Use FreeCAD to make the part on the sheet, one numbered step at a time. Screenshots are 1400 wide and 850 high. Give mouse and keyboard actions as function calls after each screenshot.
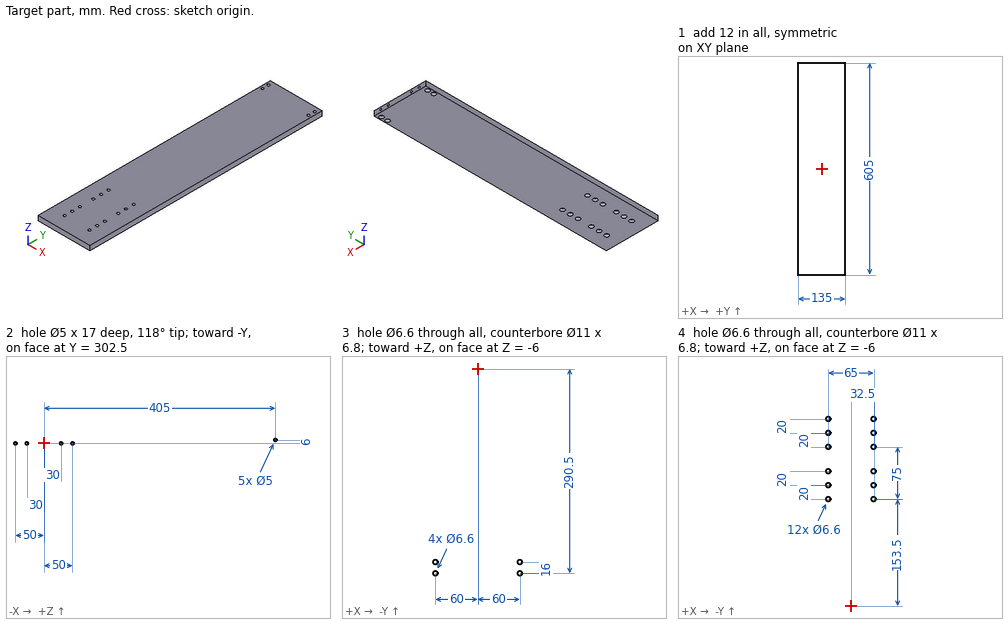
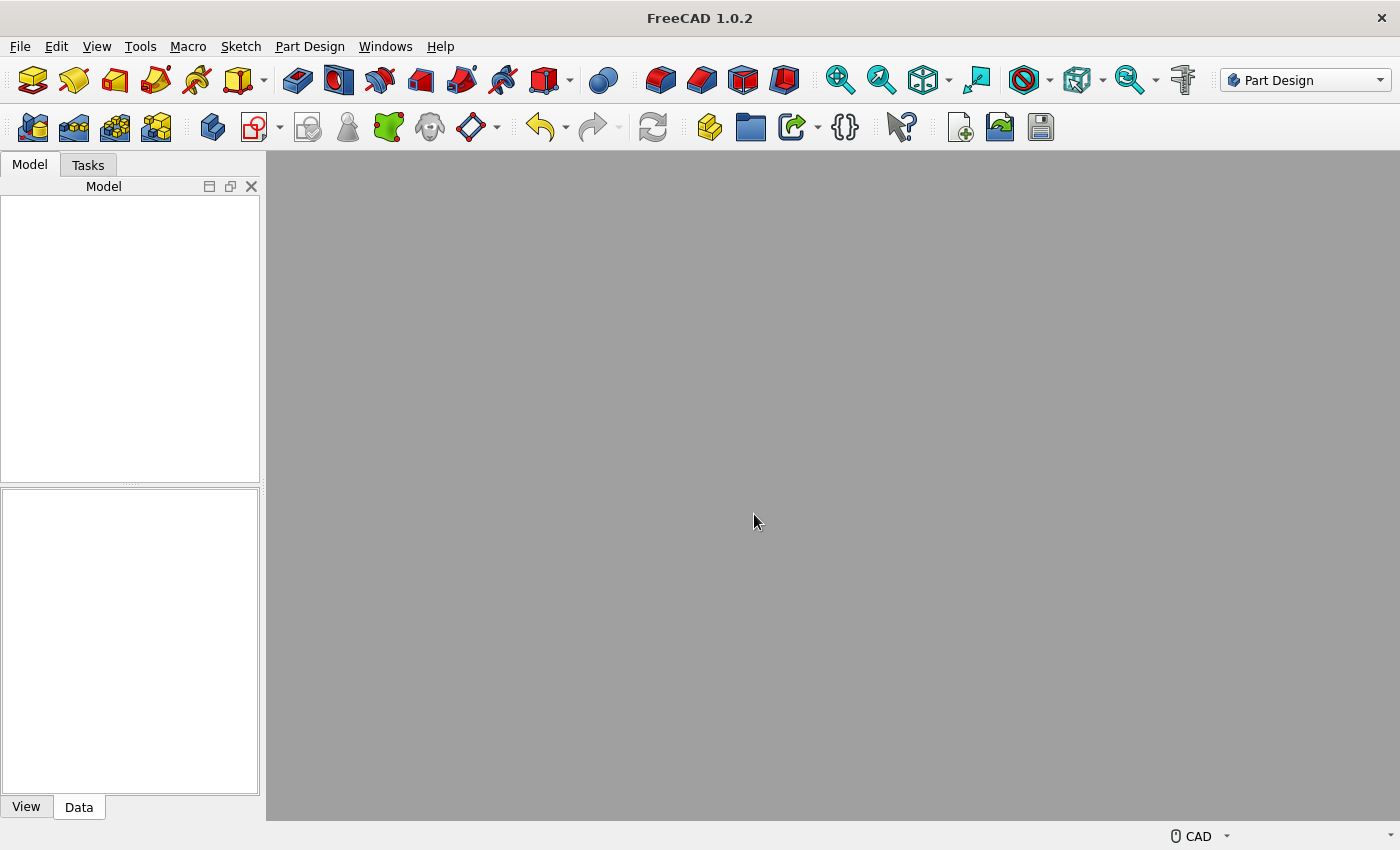
click(959, 128)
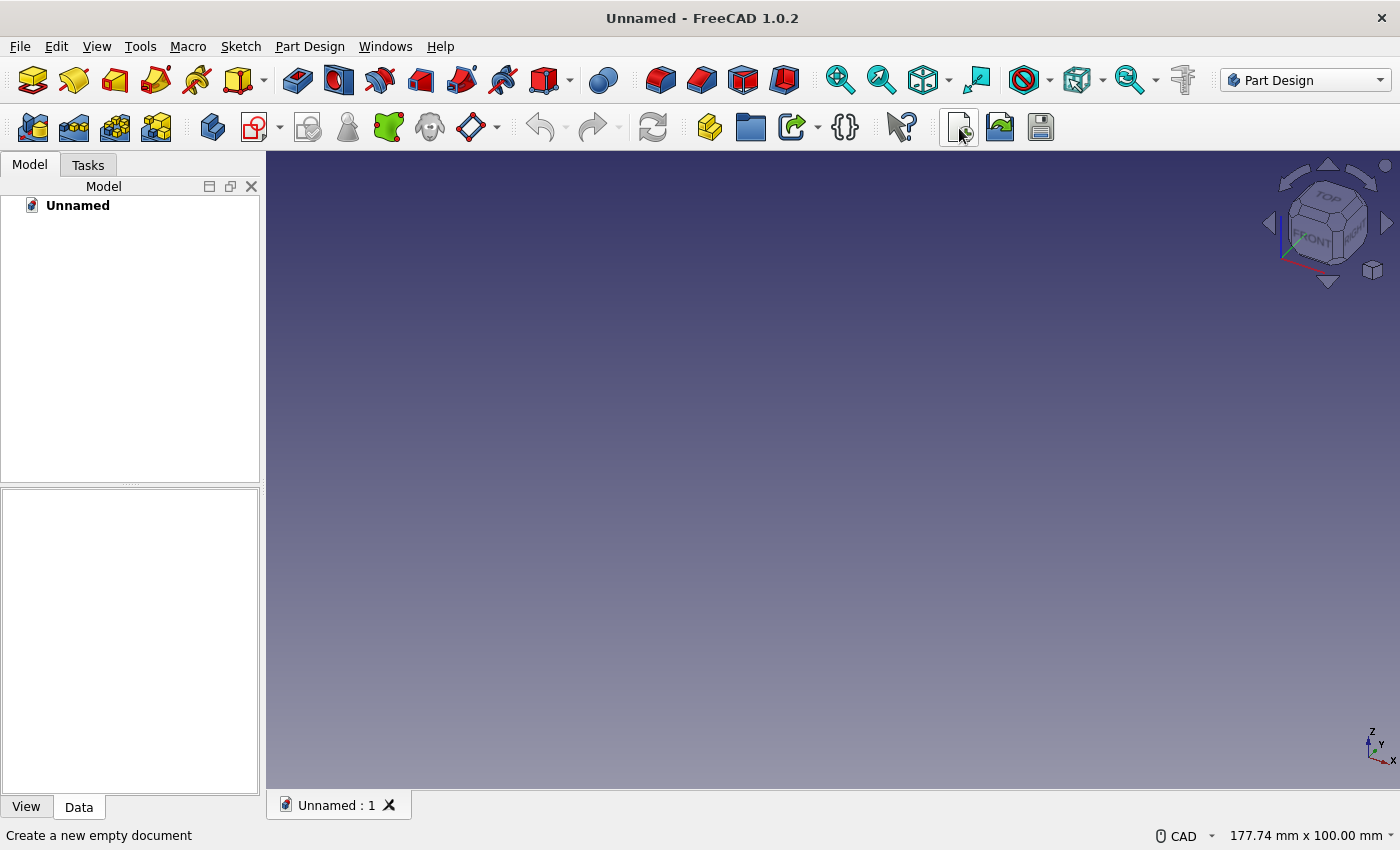
click(254, 128)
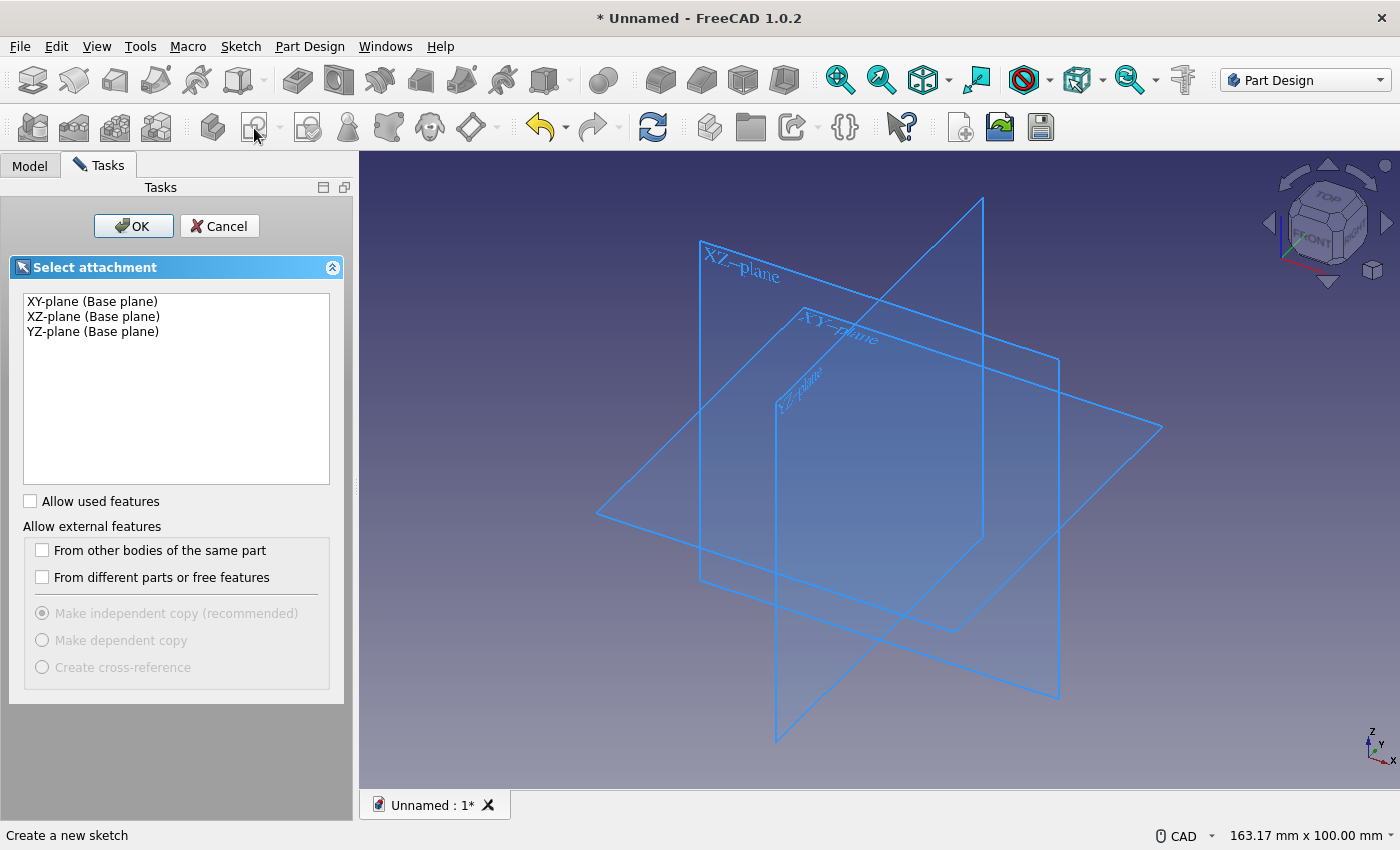
click(84, 302)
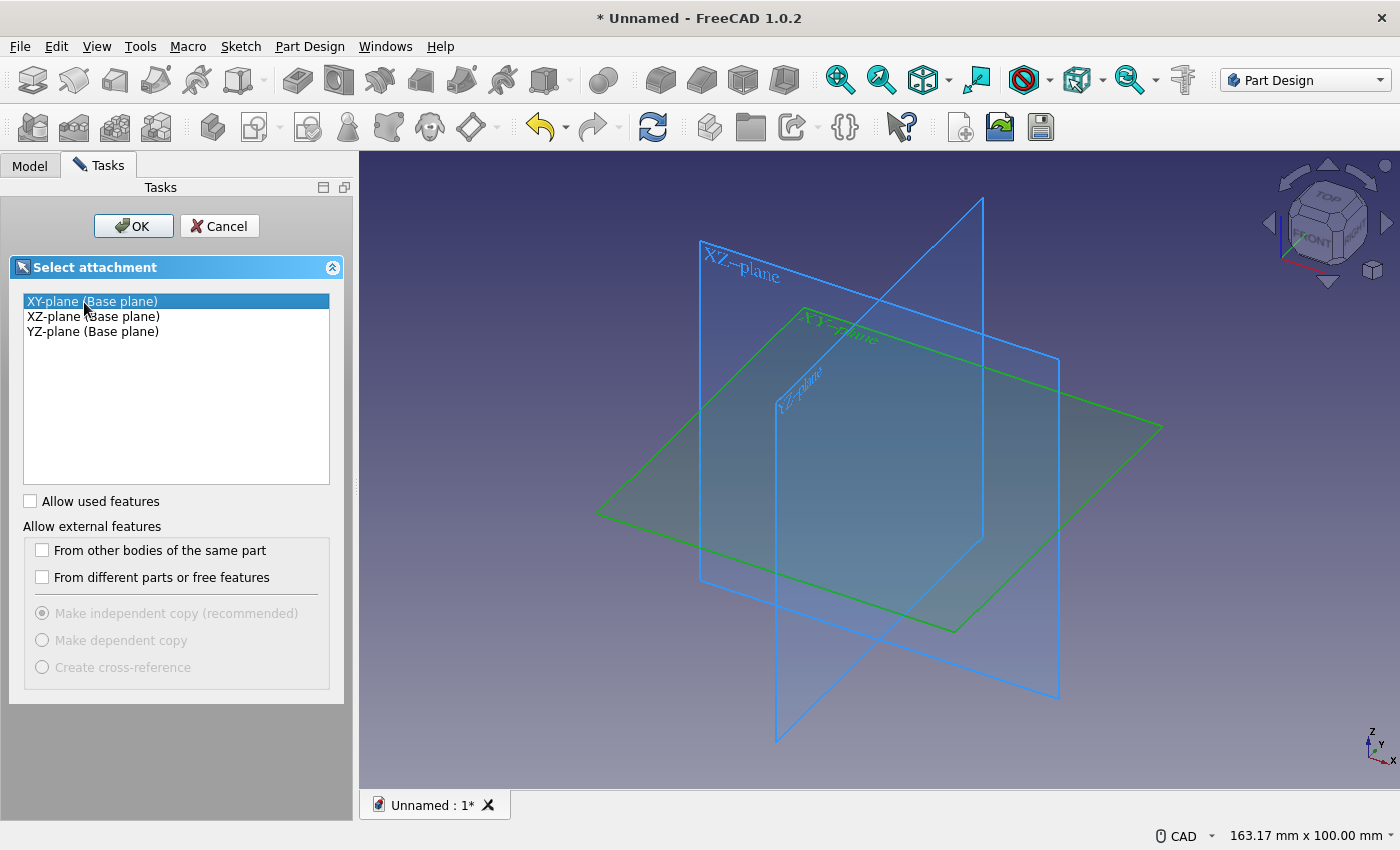
click(134, 226)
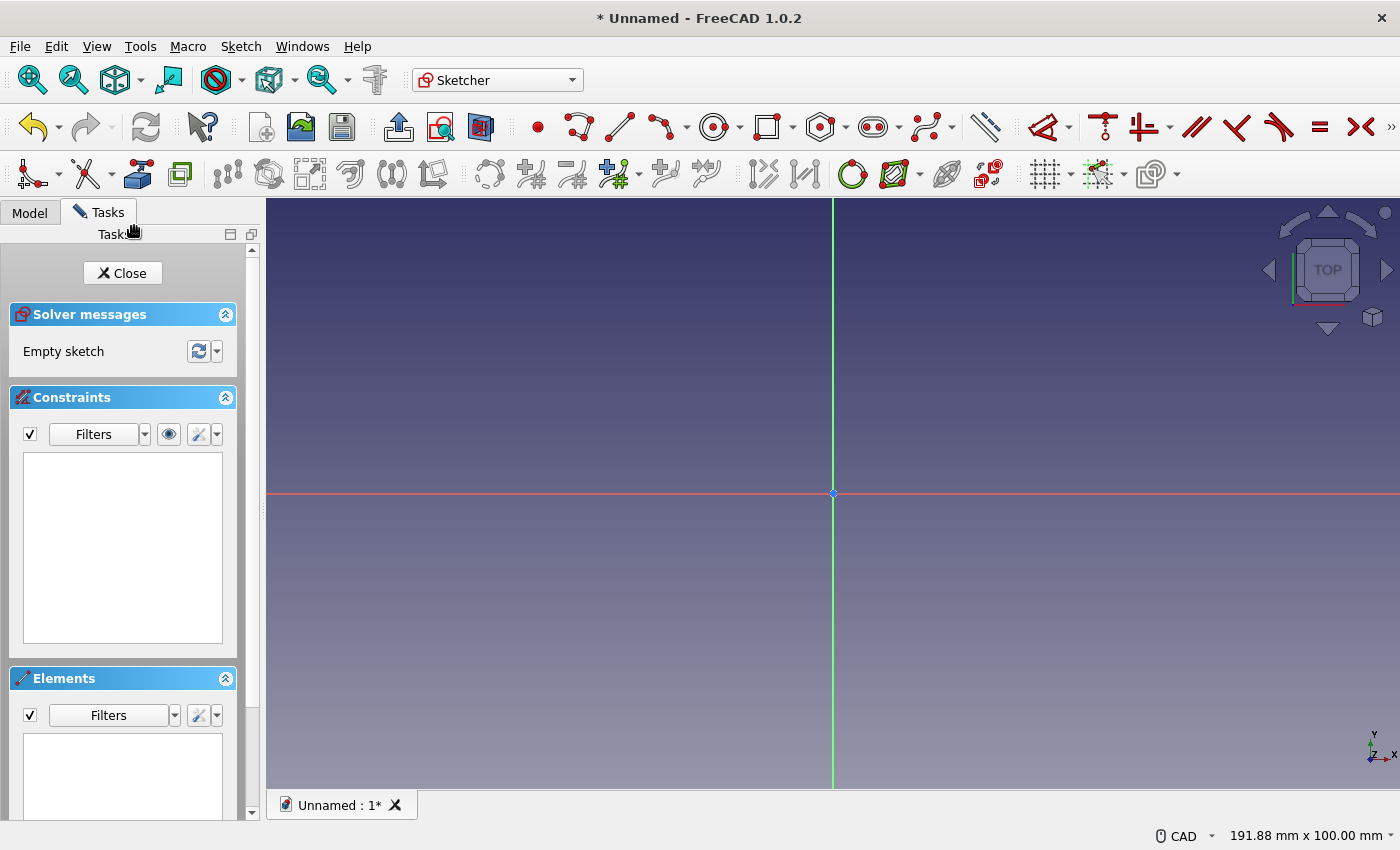
scroll(756, 494, down, 11)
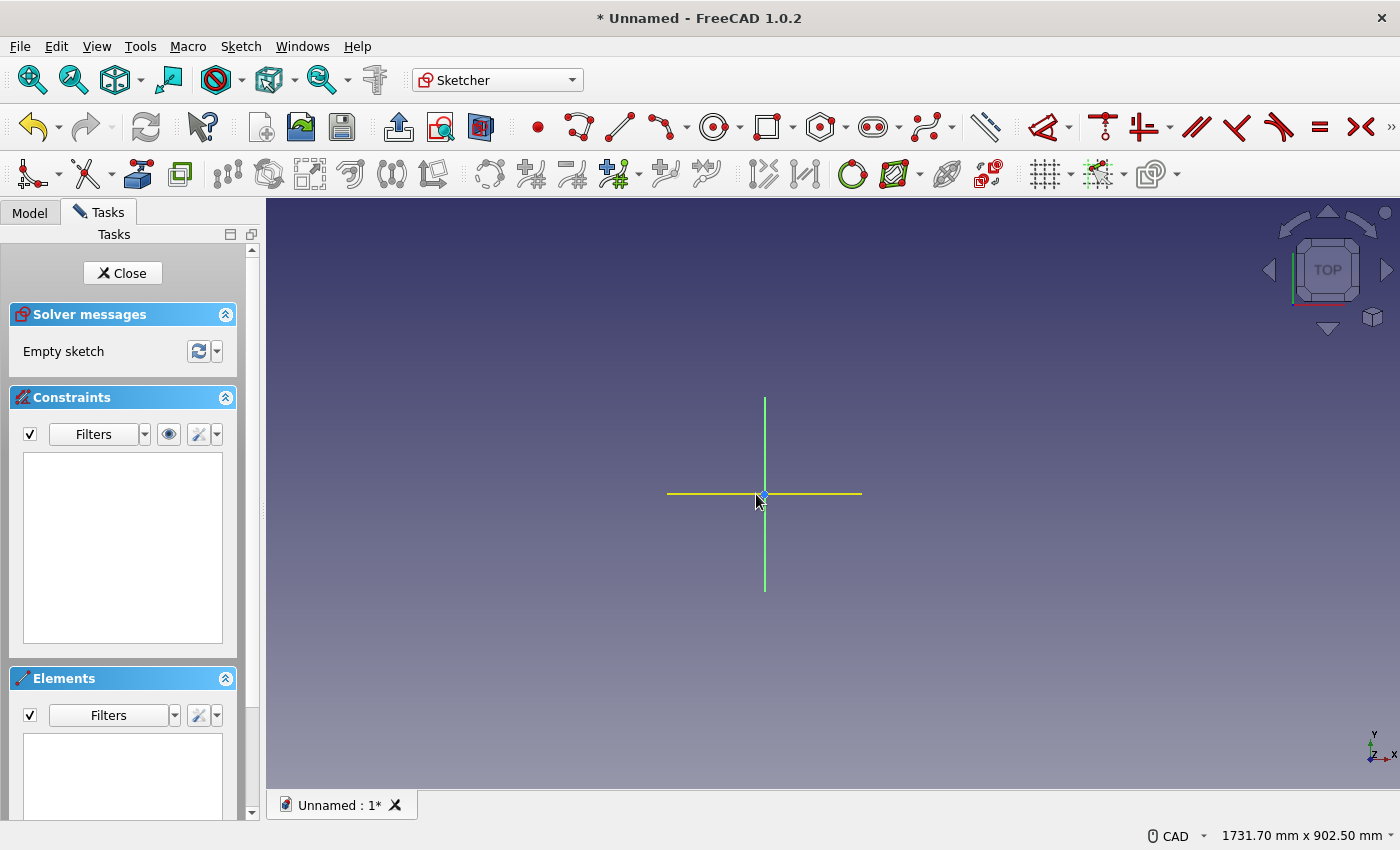
key(g)
key(v)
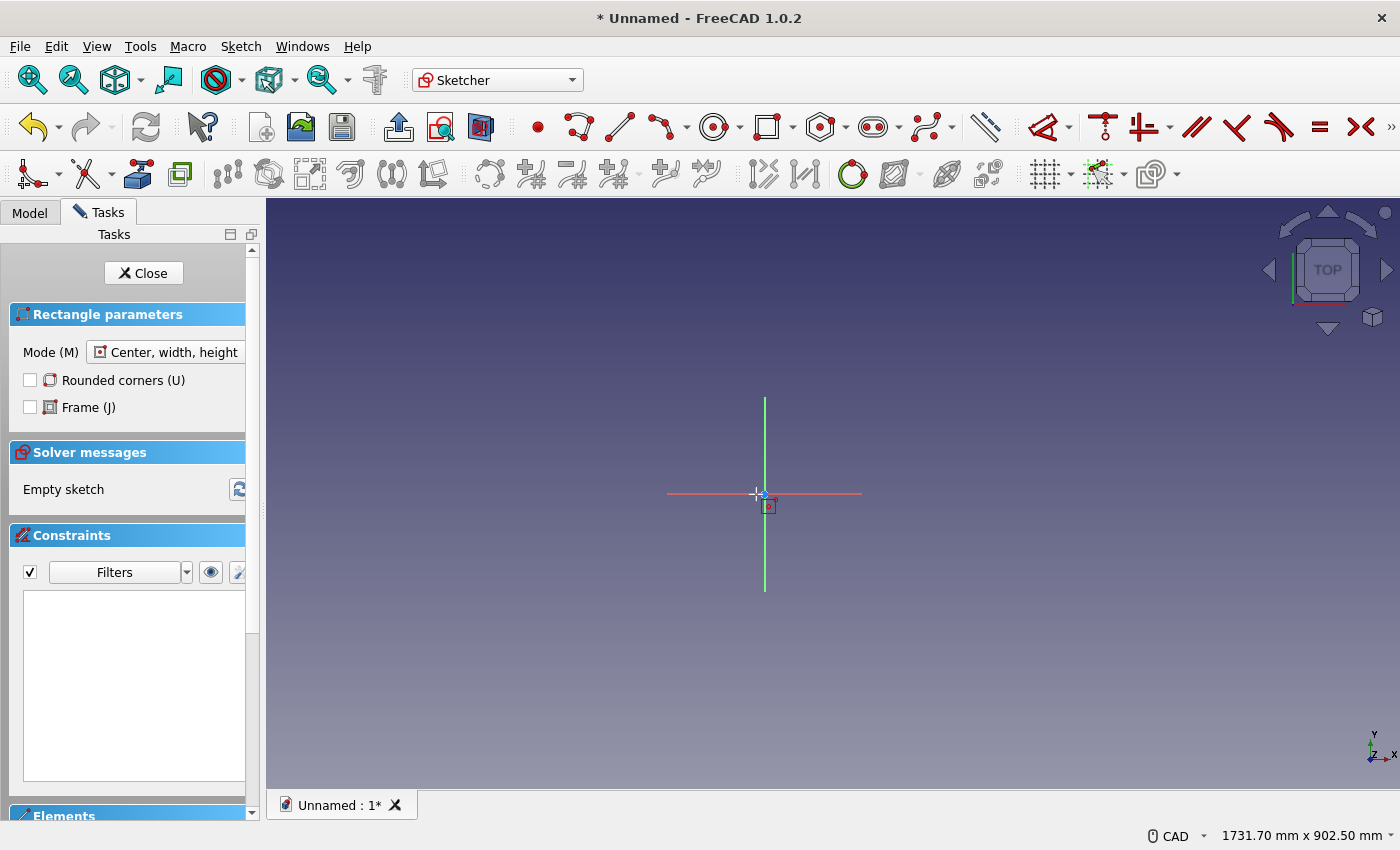
click(765, 494)
move(809, 296)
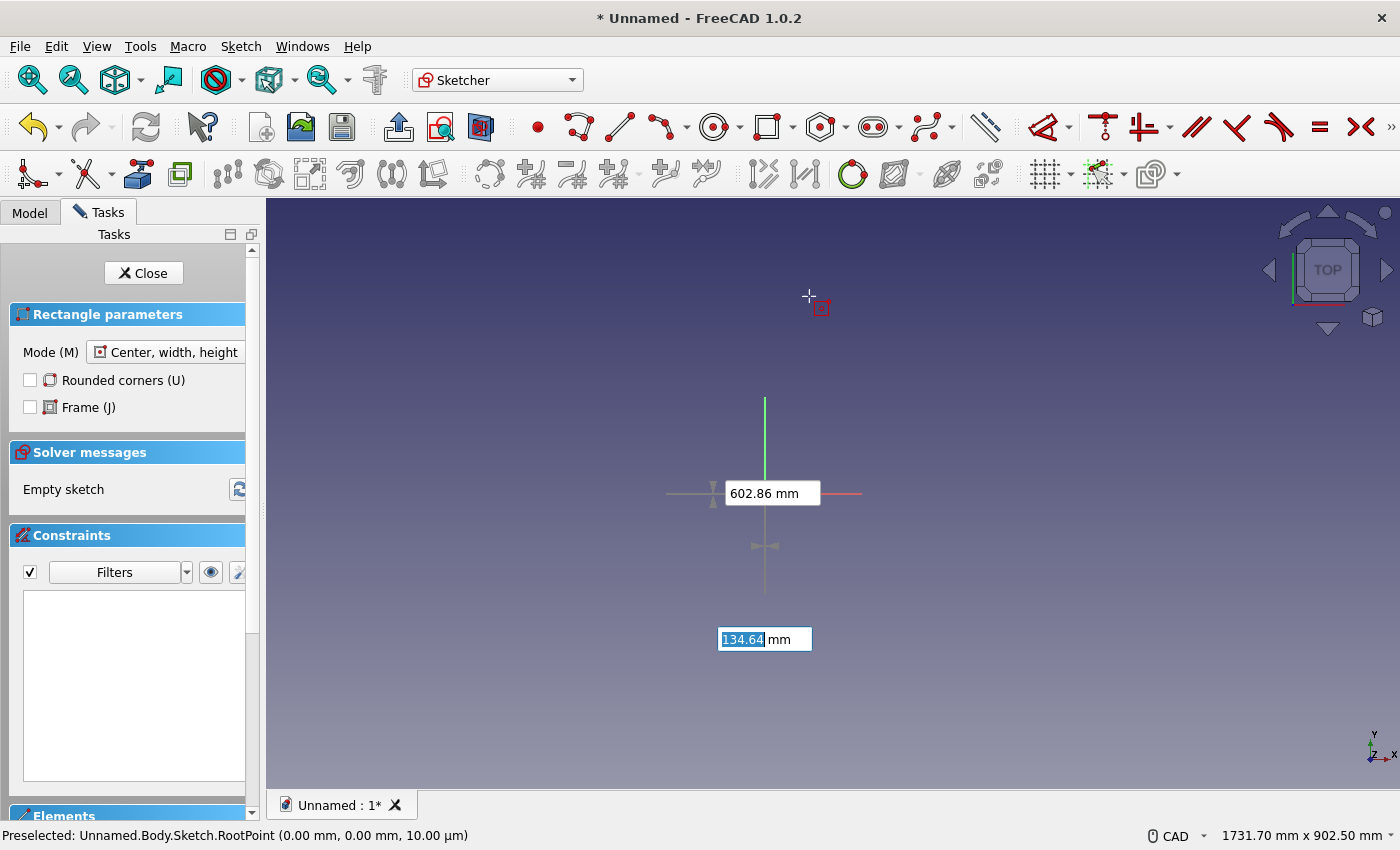
text(135)
key(Tab)
text(605)
key(Return)
key(Escape)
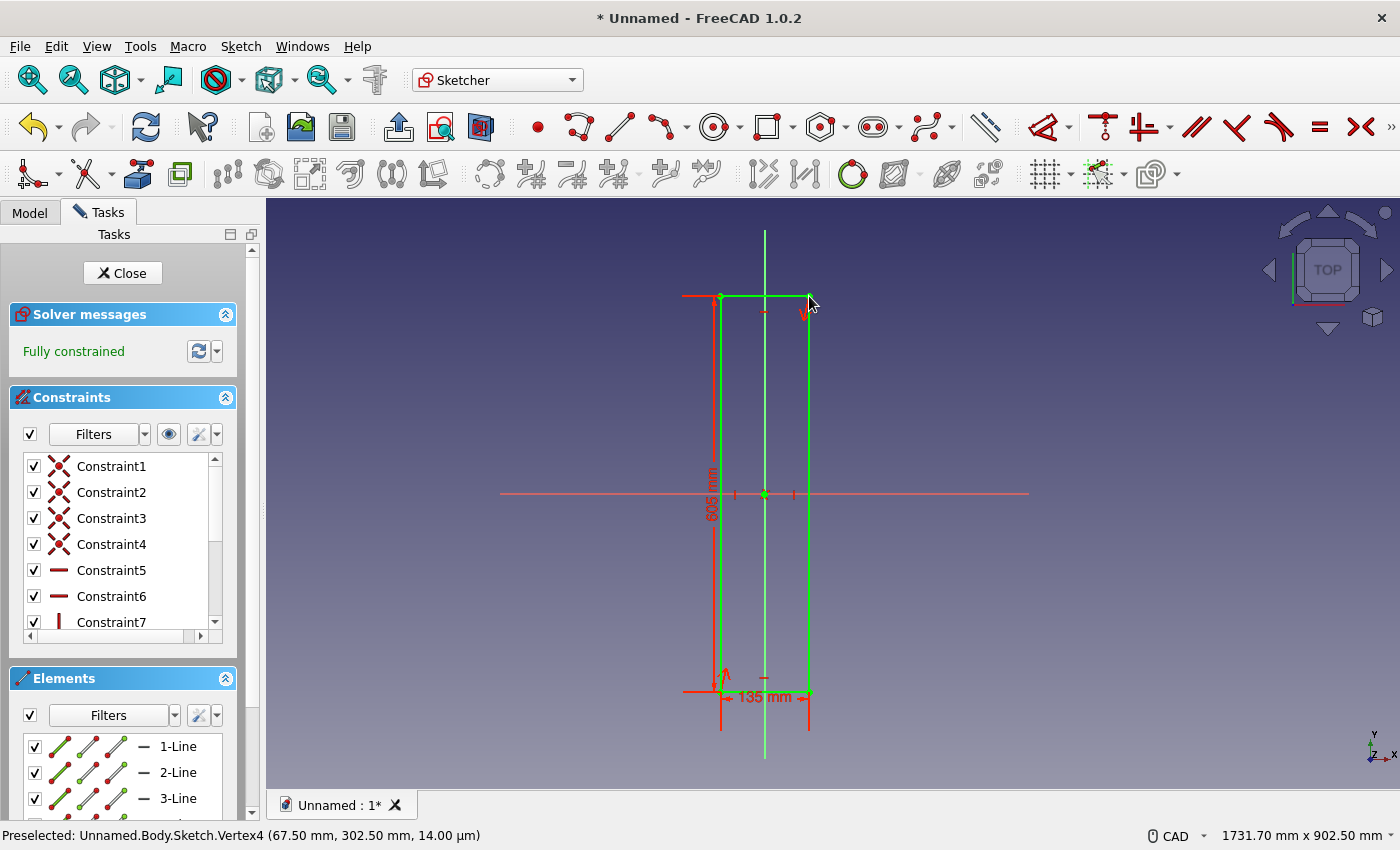
click(123, 273)